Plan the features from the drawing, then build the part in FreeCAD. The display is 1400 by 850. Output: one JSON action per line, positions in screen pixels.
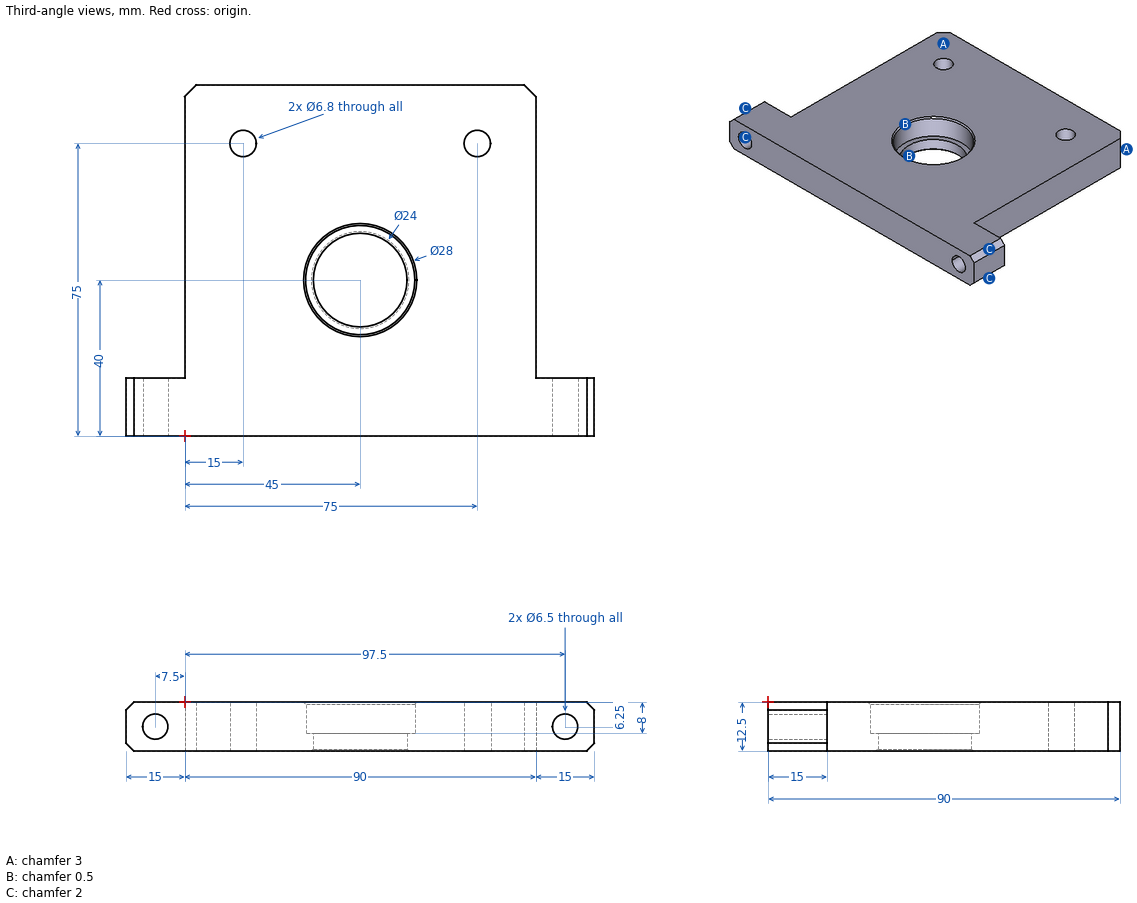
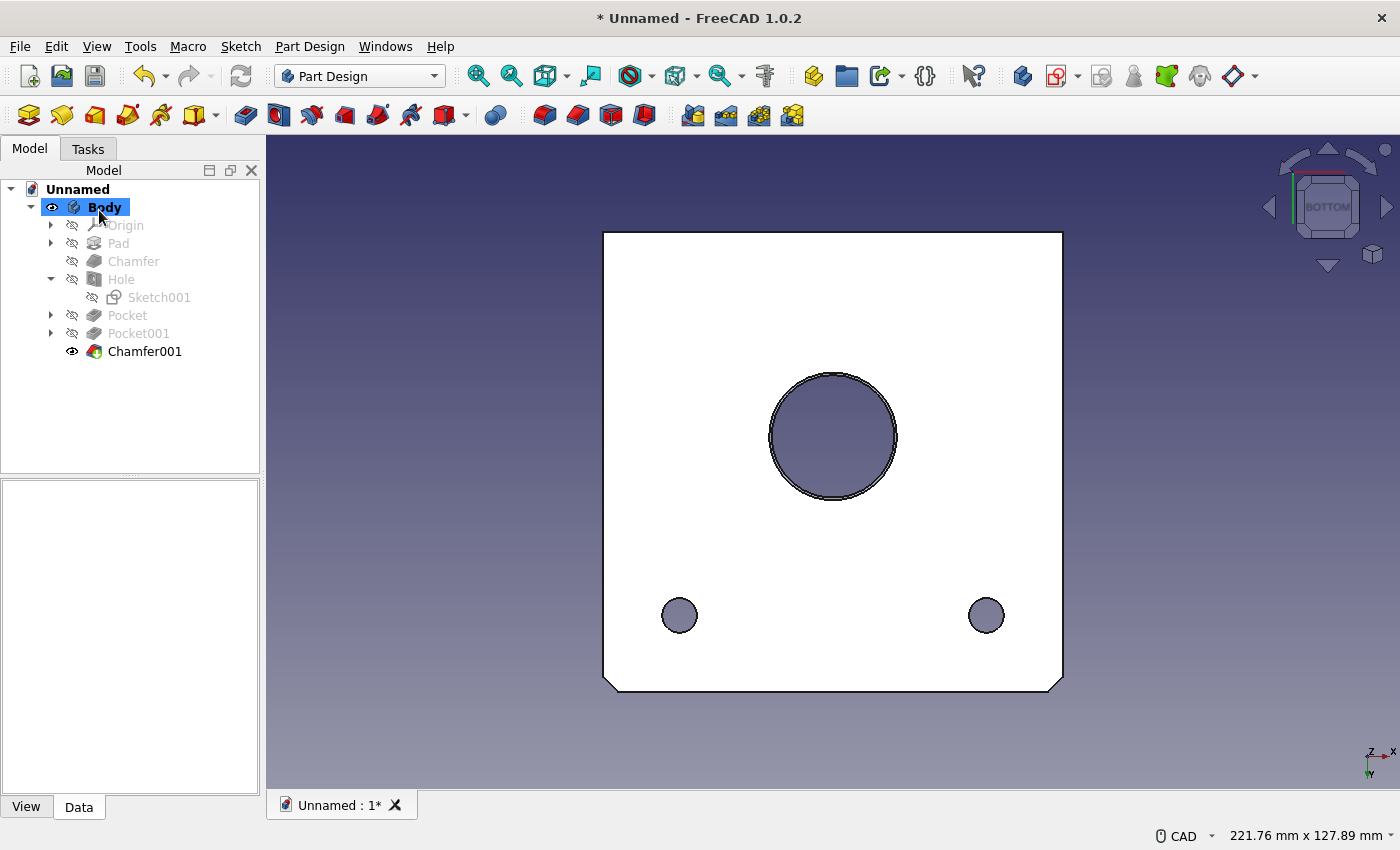
{"action": "key", "text": "0"}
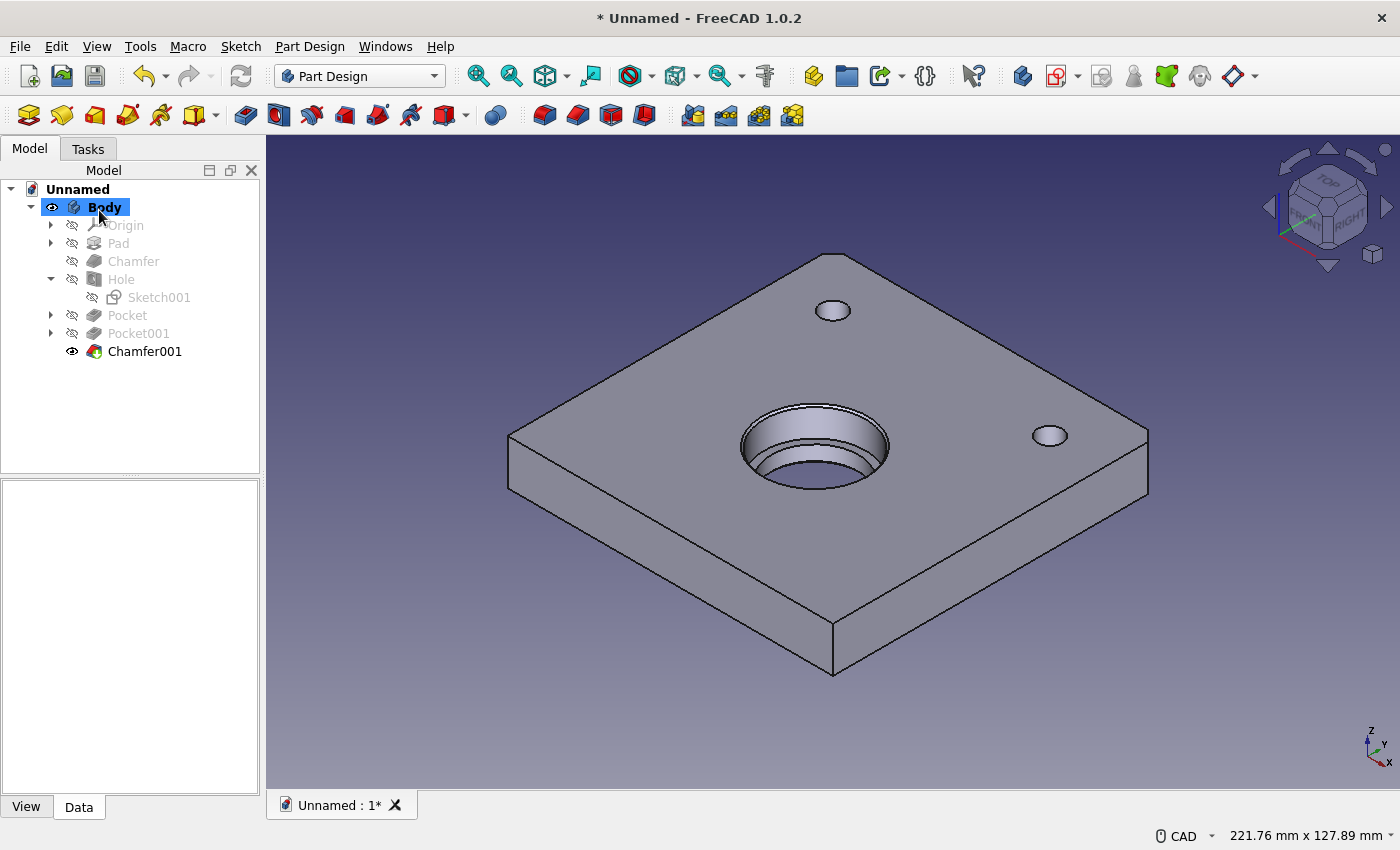
{"action": "left_click", "coordinate": [990, 558]}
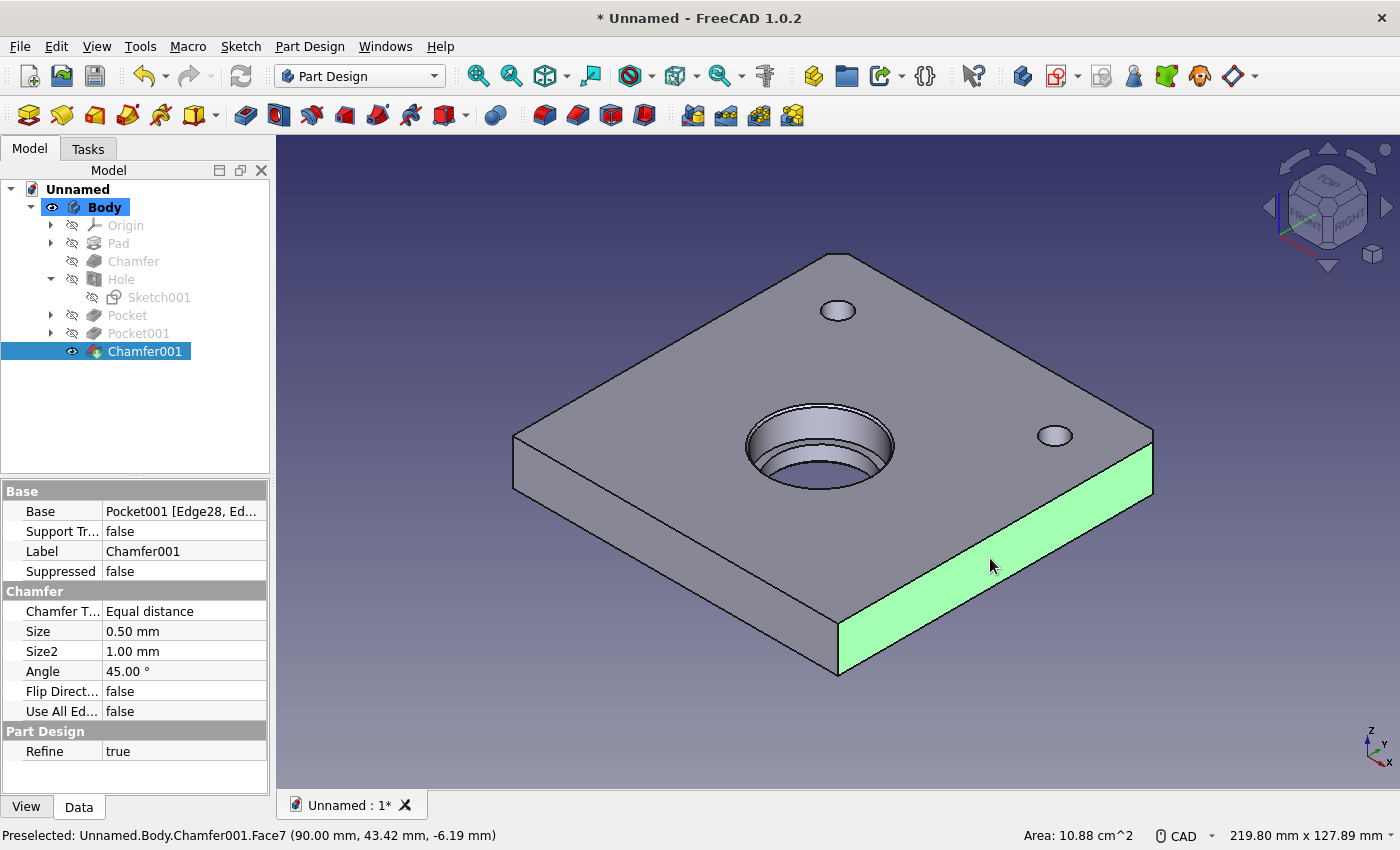
{"action": "left_click", "coordinate": [1056, 76]}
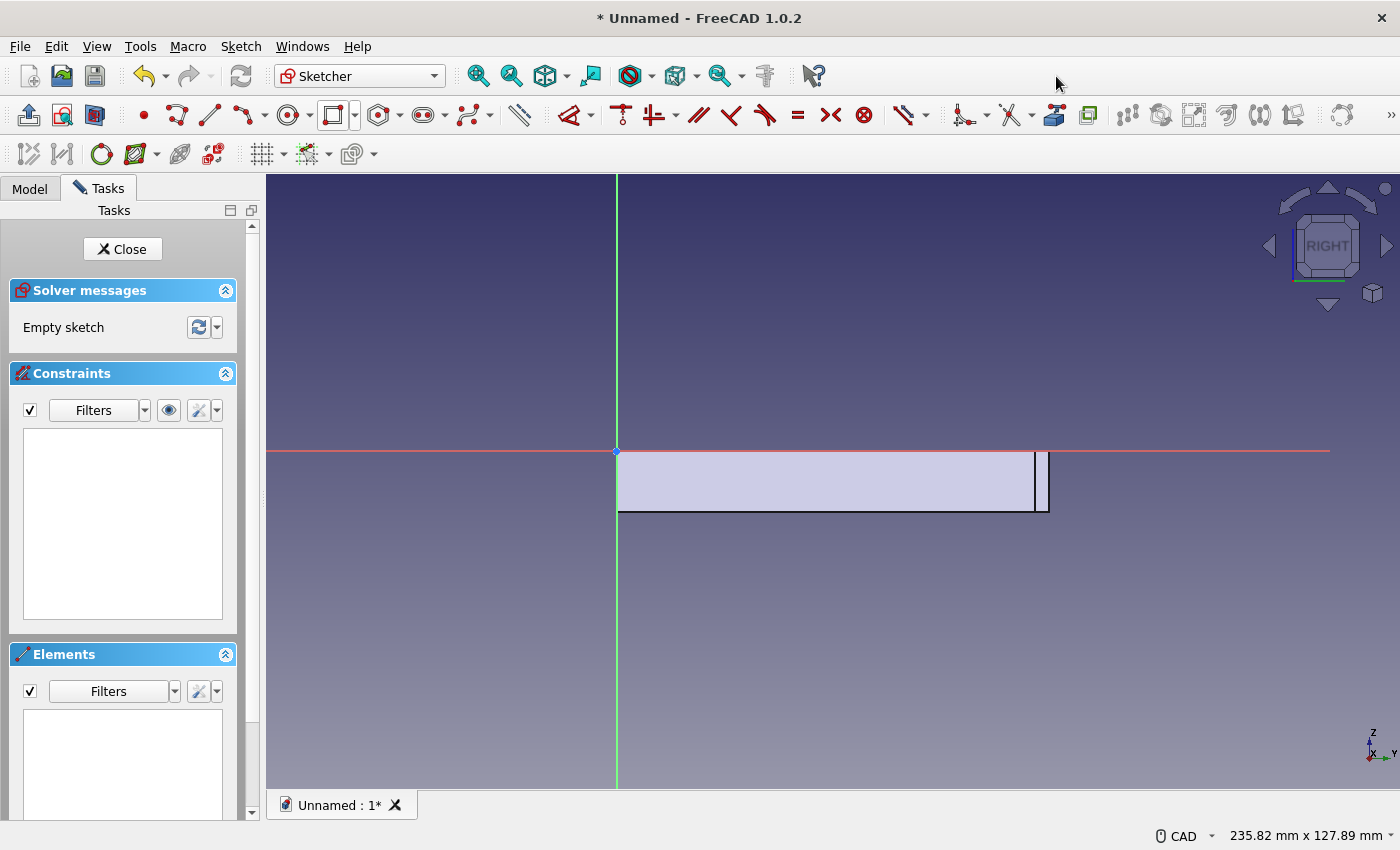
{"action": "scroll", "coordinate": [631, 481], "scroll_direction": "up", "scroll_amount": 9}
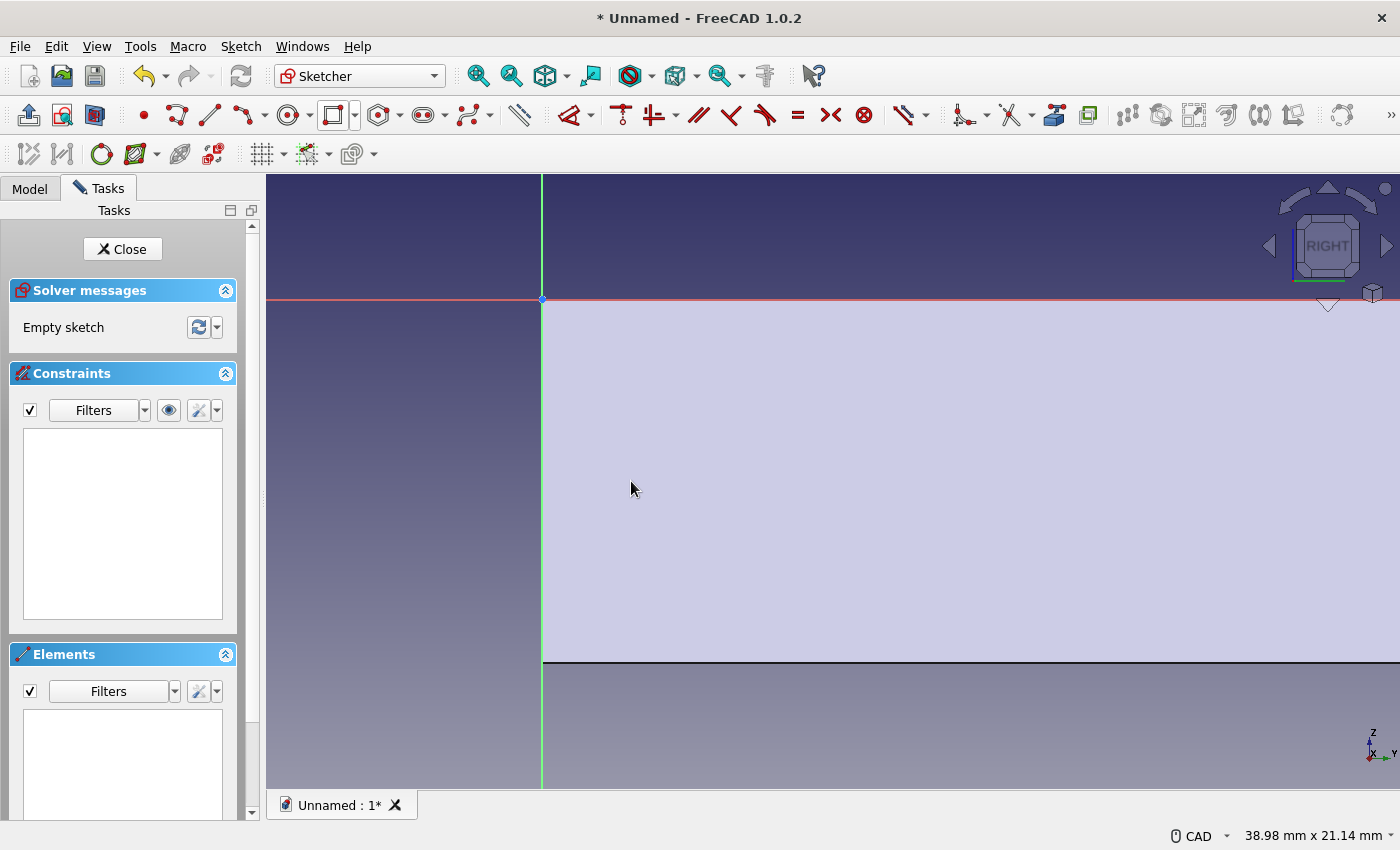
{"action": "left_click", "coordinate": [332, 116]}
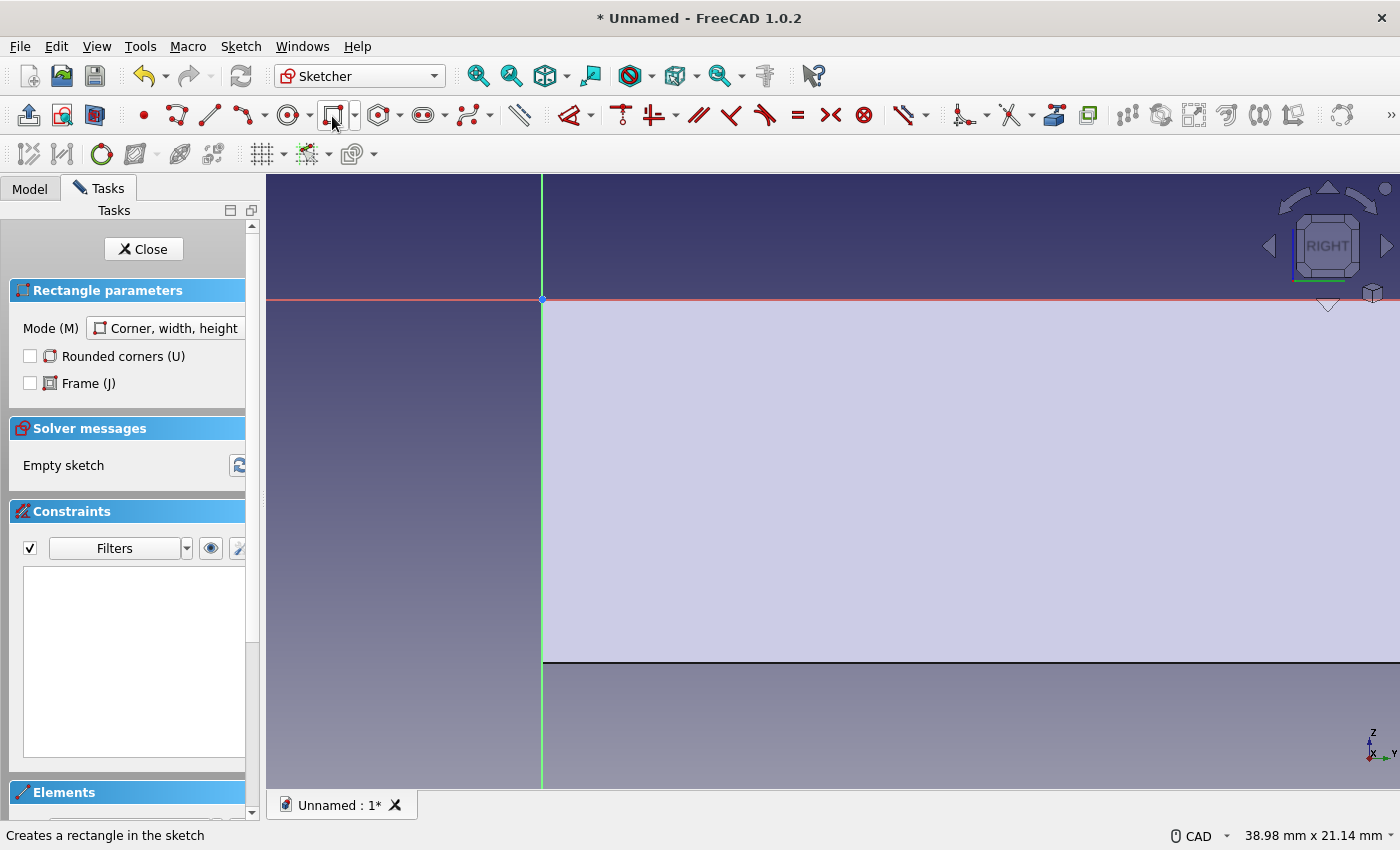
{"action": "left_click", "coordinate": [542, 300]}
{"action": "left_click", "coordinate": [979, 663]}
{"action": "key", "text": "Escape"}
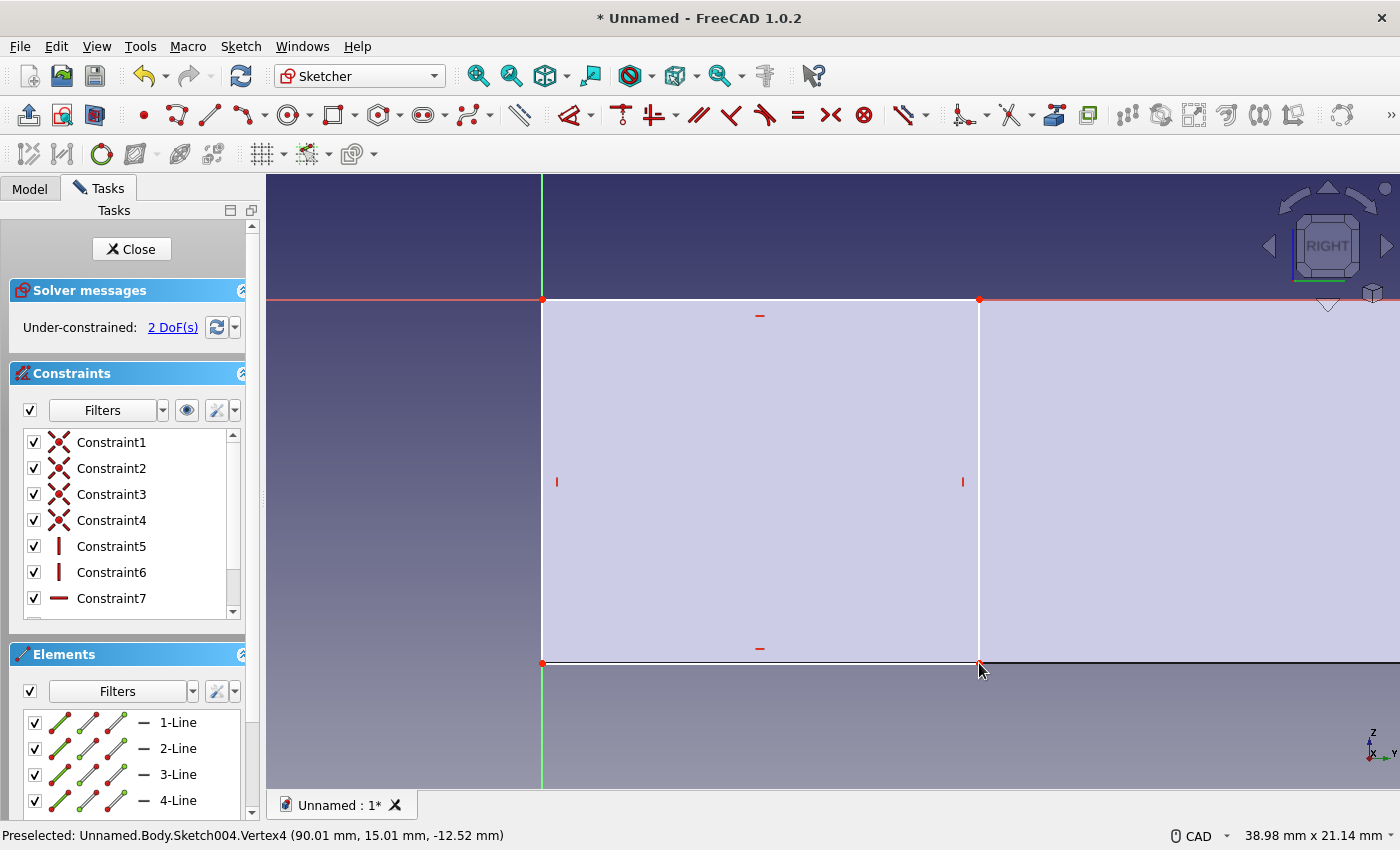
{"action": "left_click", "coordinate": [568, 116]}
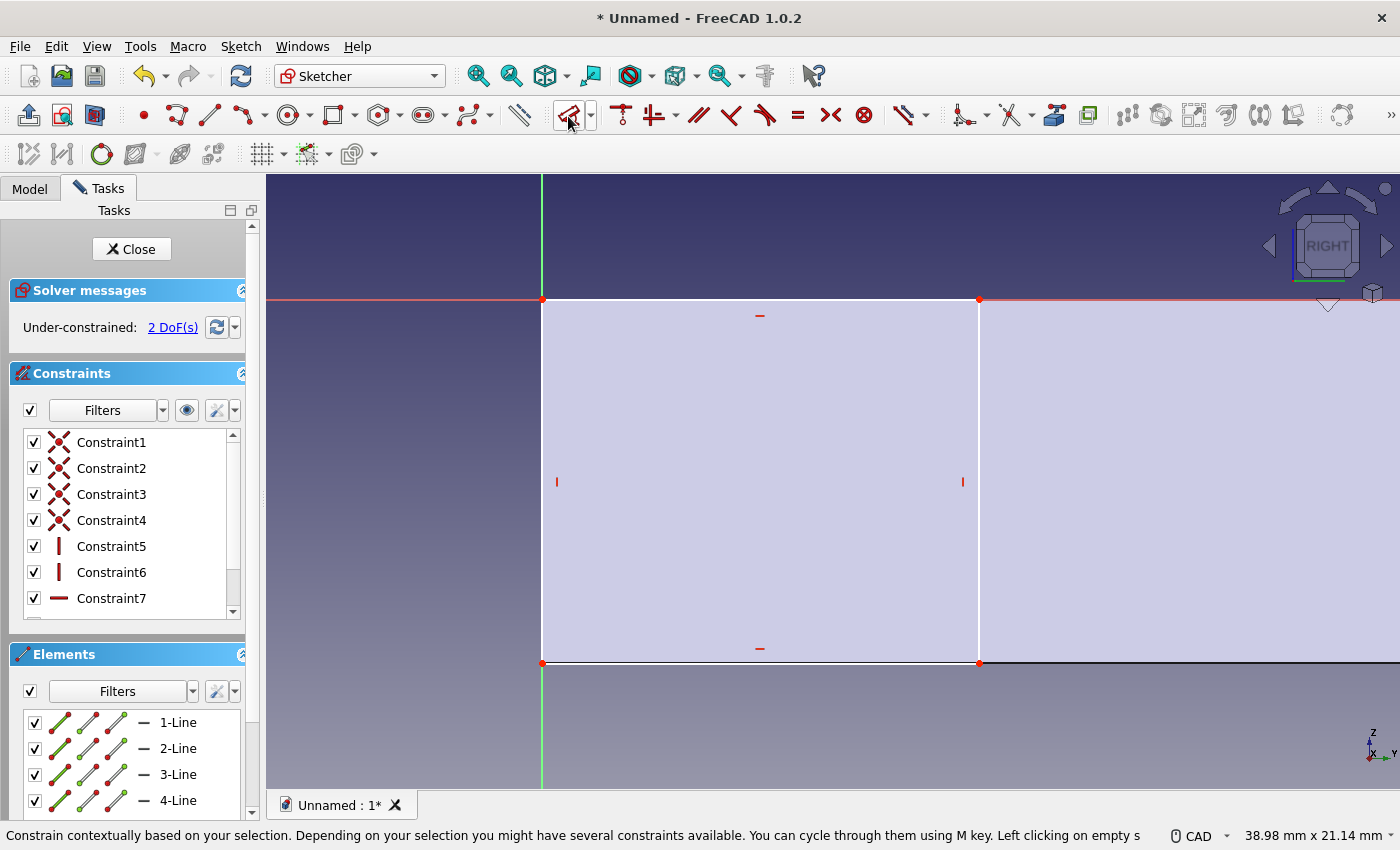
{"action": "left_click", "coordinate": [673, 664]}
{"action": "left_click", "coordinate": [761, 698]}